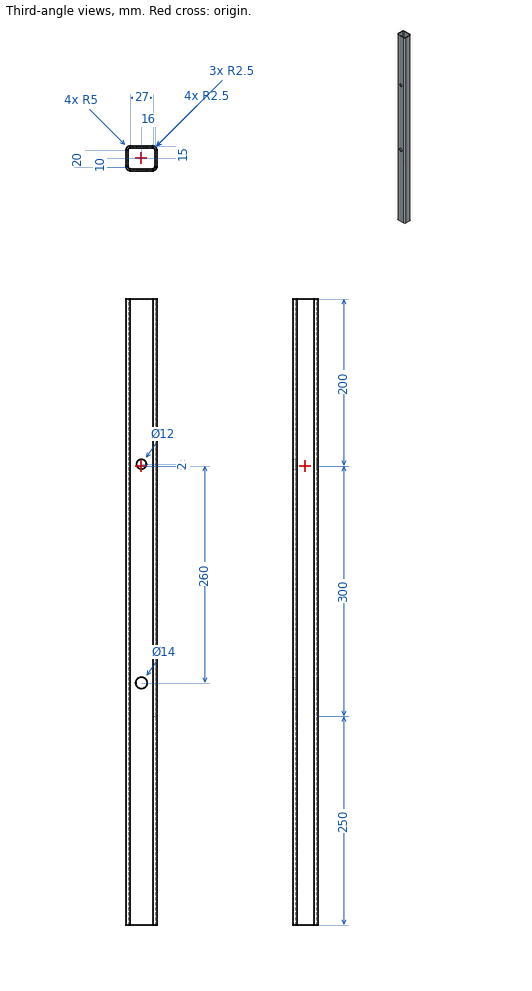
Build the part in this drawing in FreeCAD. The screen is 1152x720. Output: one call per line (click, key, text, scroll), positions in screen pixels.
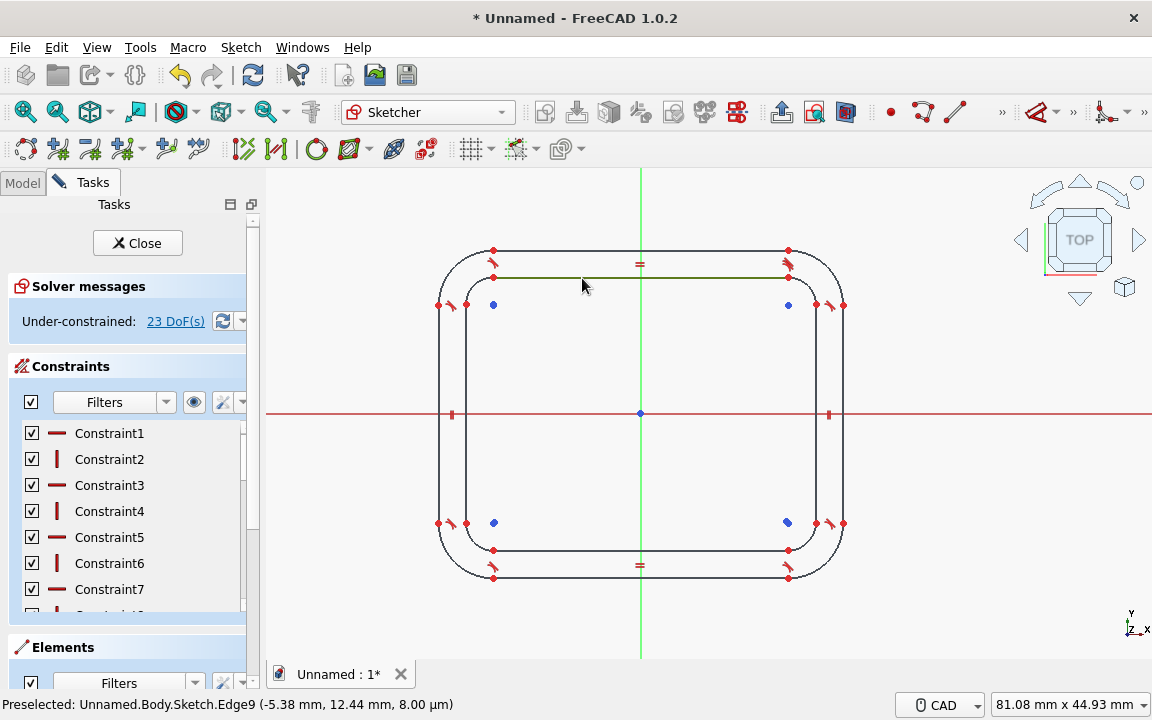
click(481, 281)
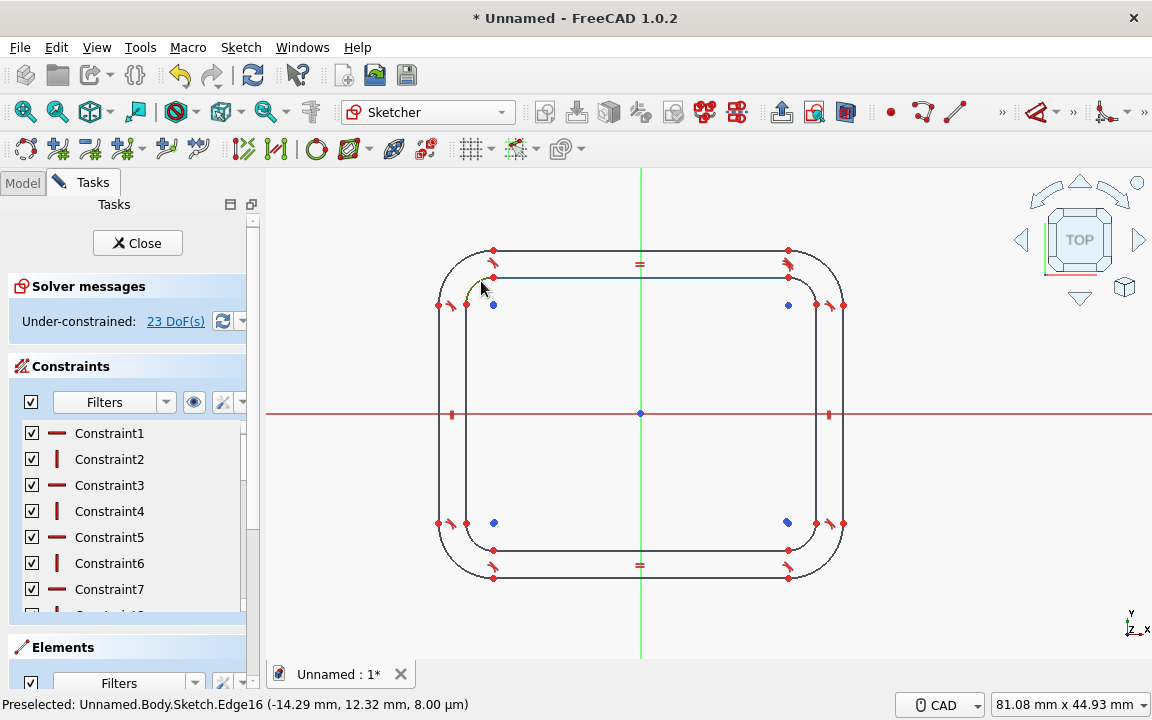
key(t)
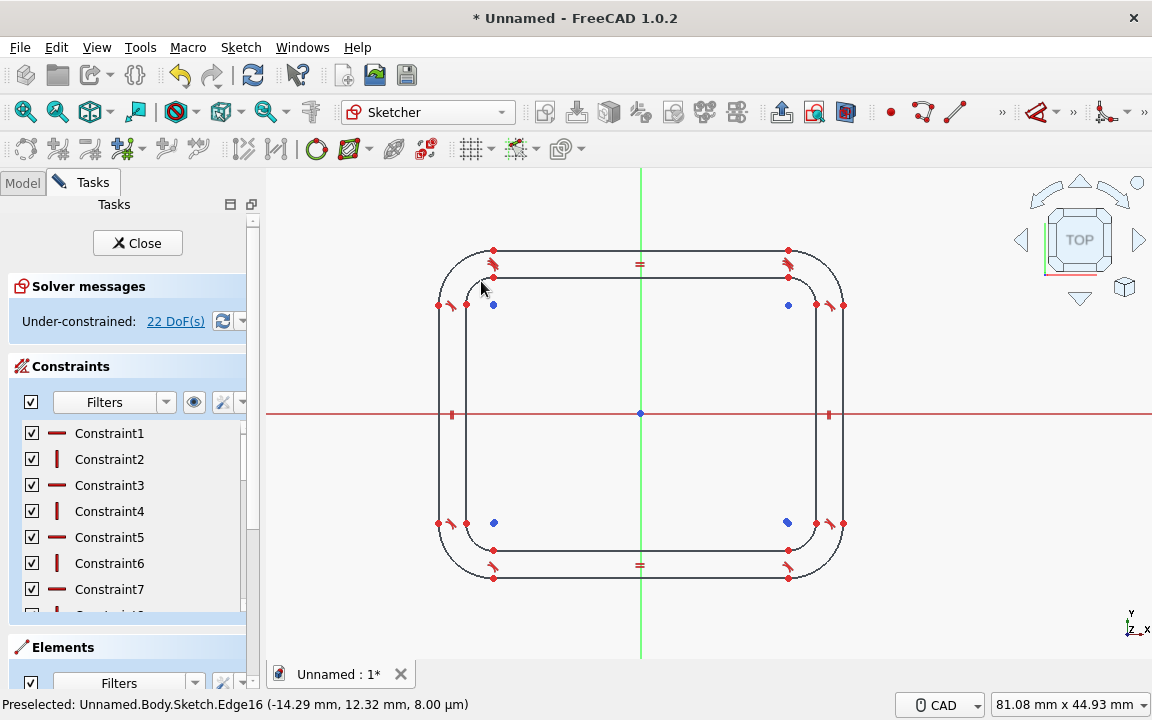
click(816, 371)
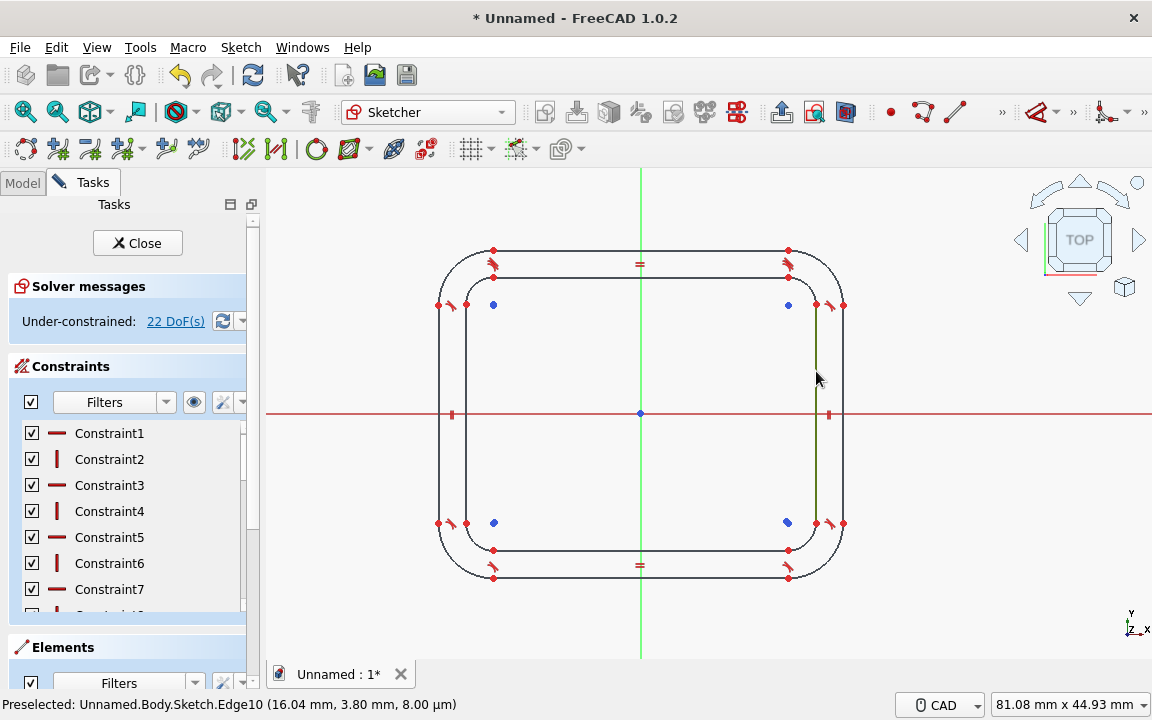
click(813, 292)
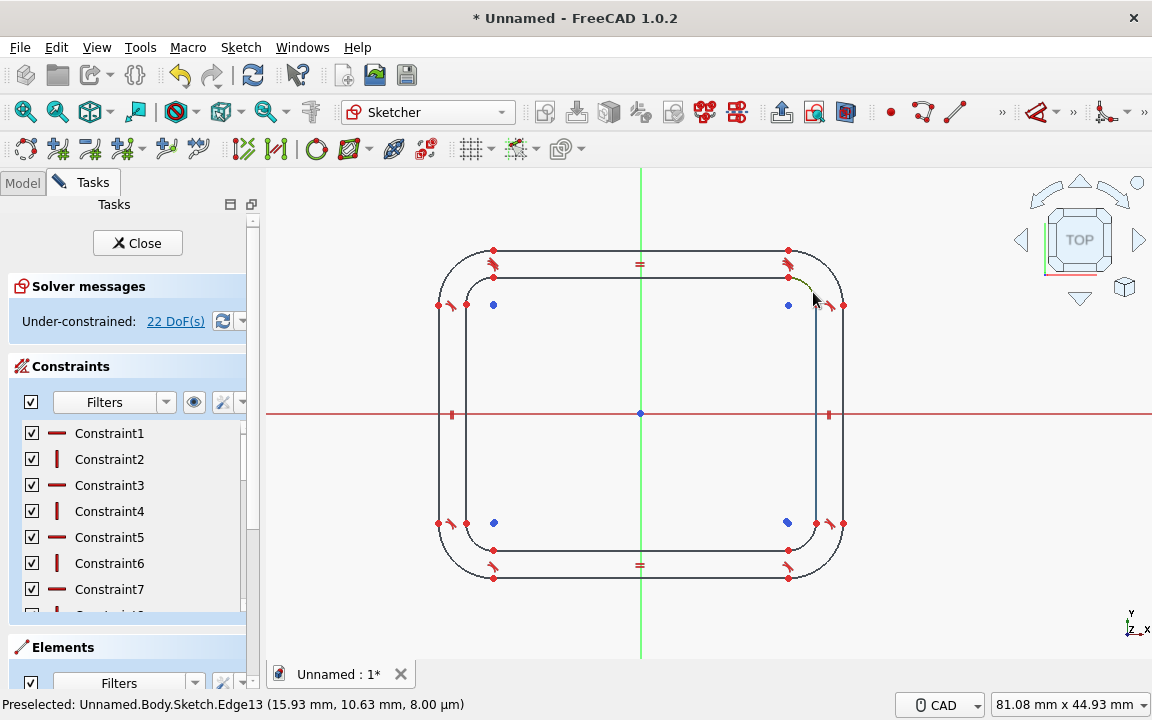
key(t)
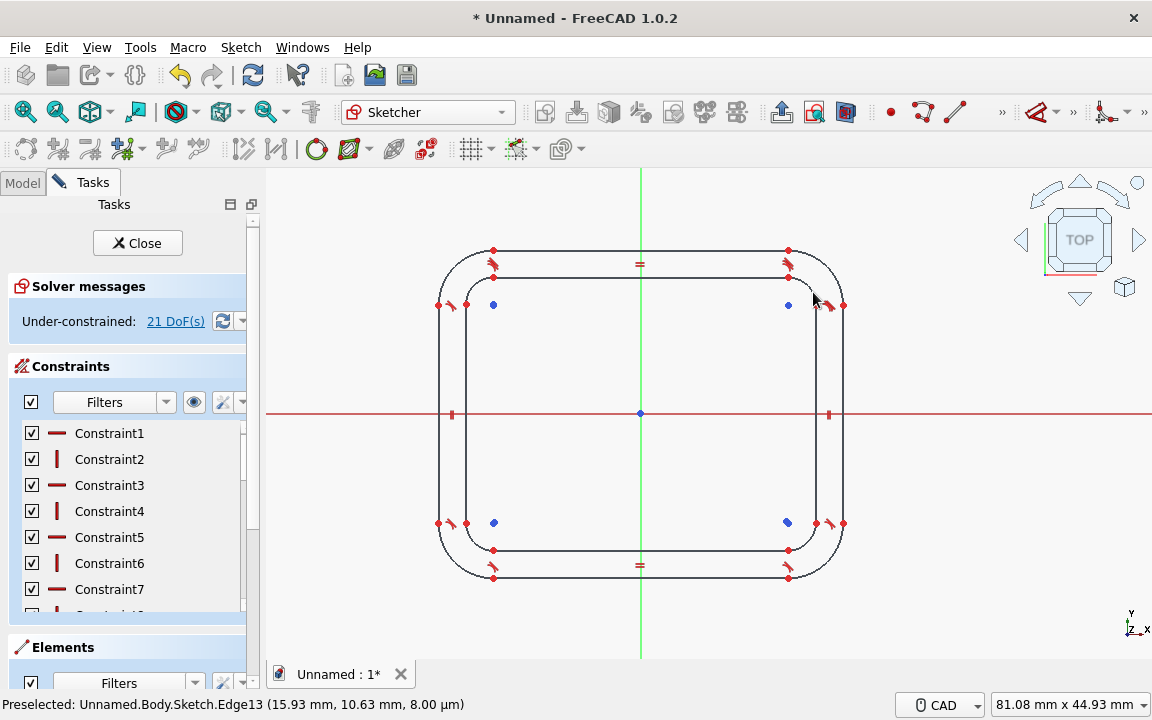
click(816, 371)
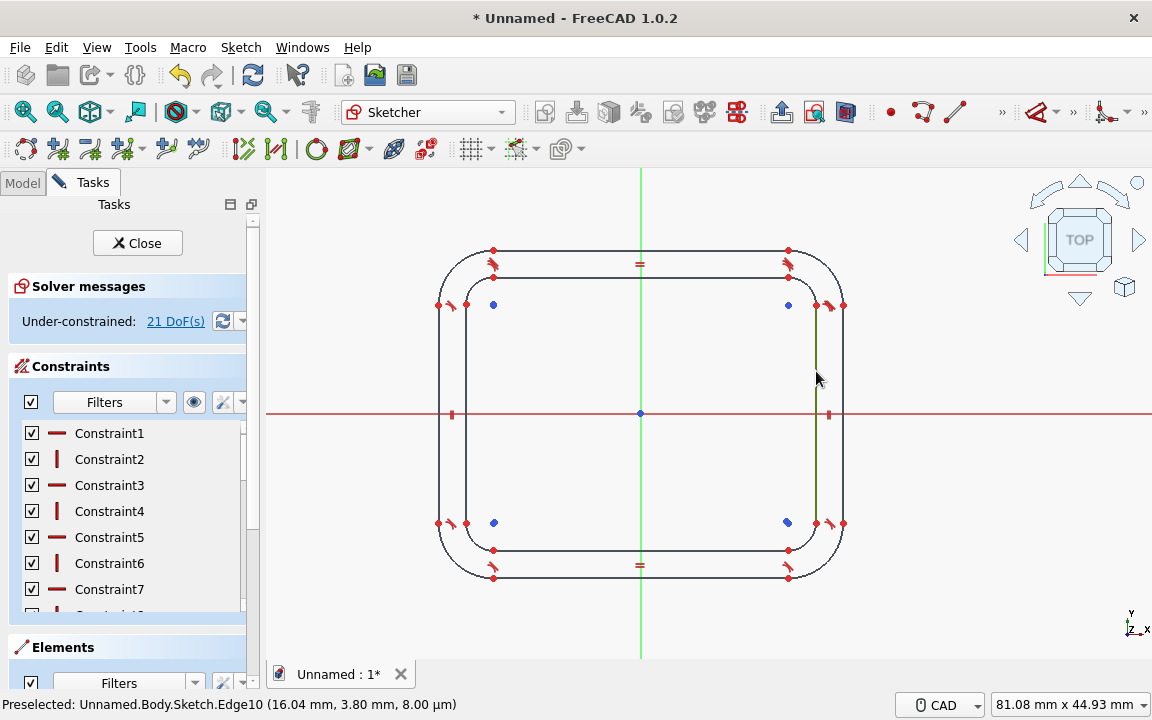
click(800, 548)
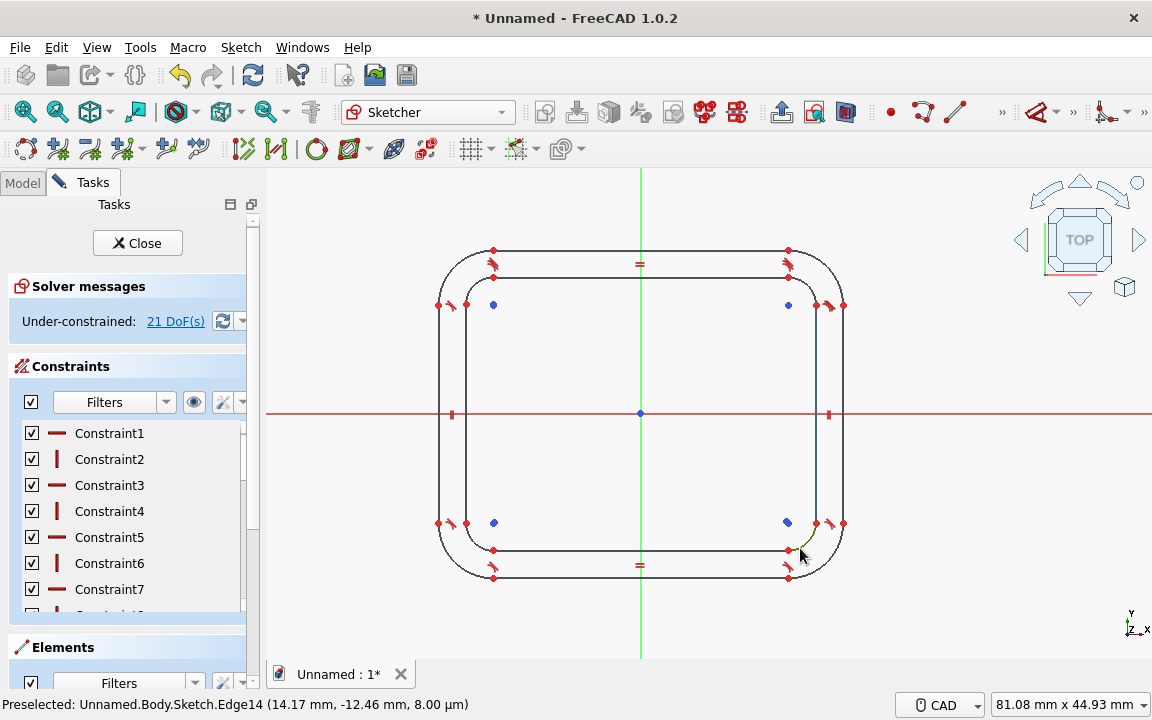
key(t)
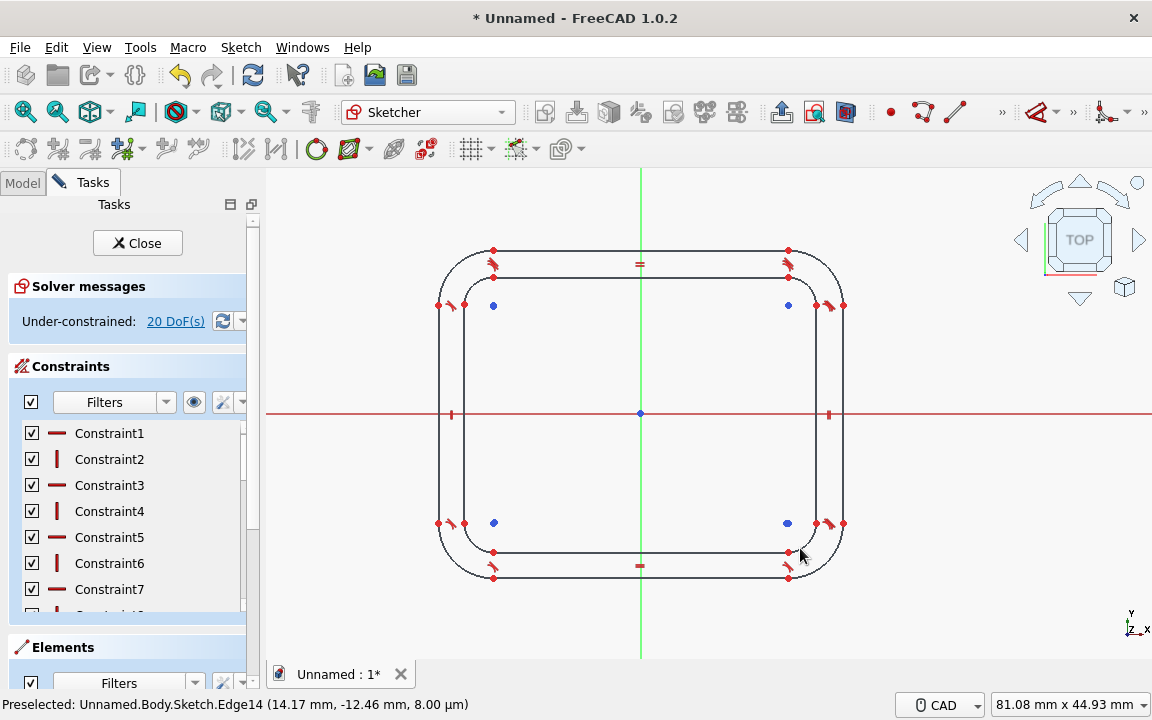
click(700, 553)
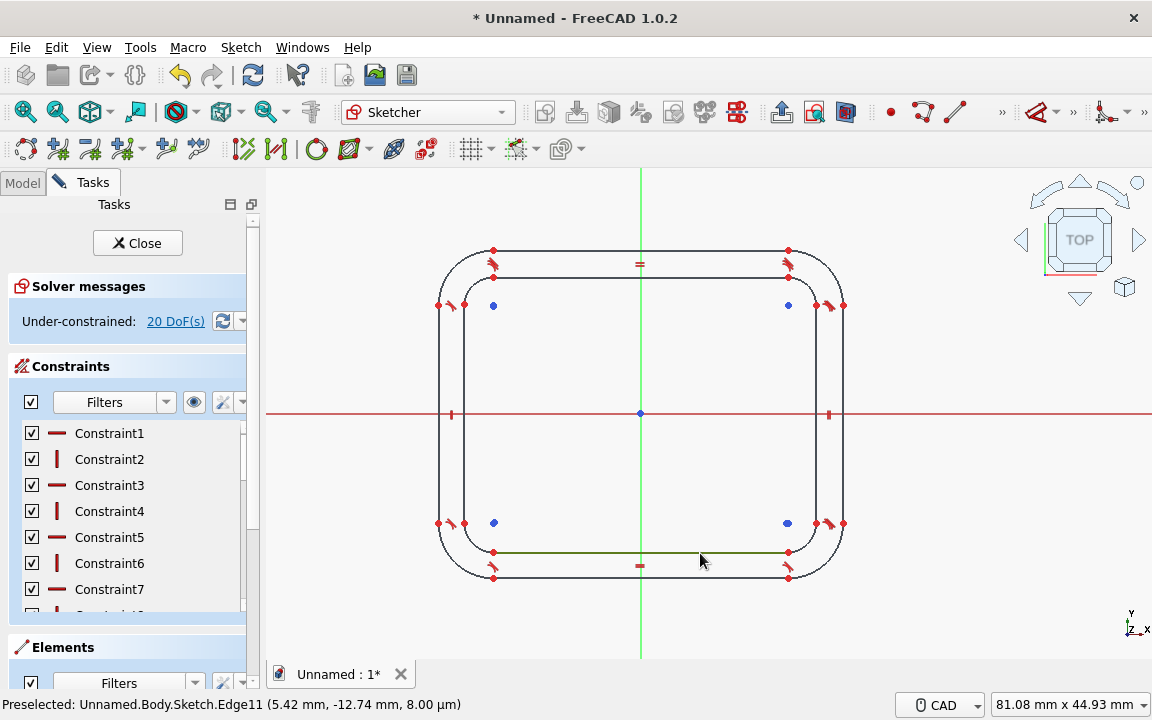
click(801, 549)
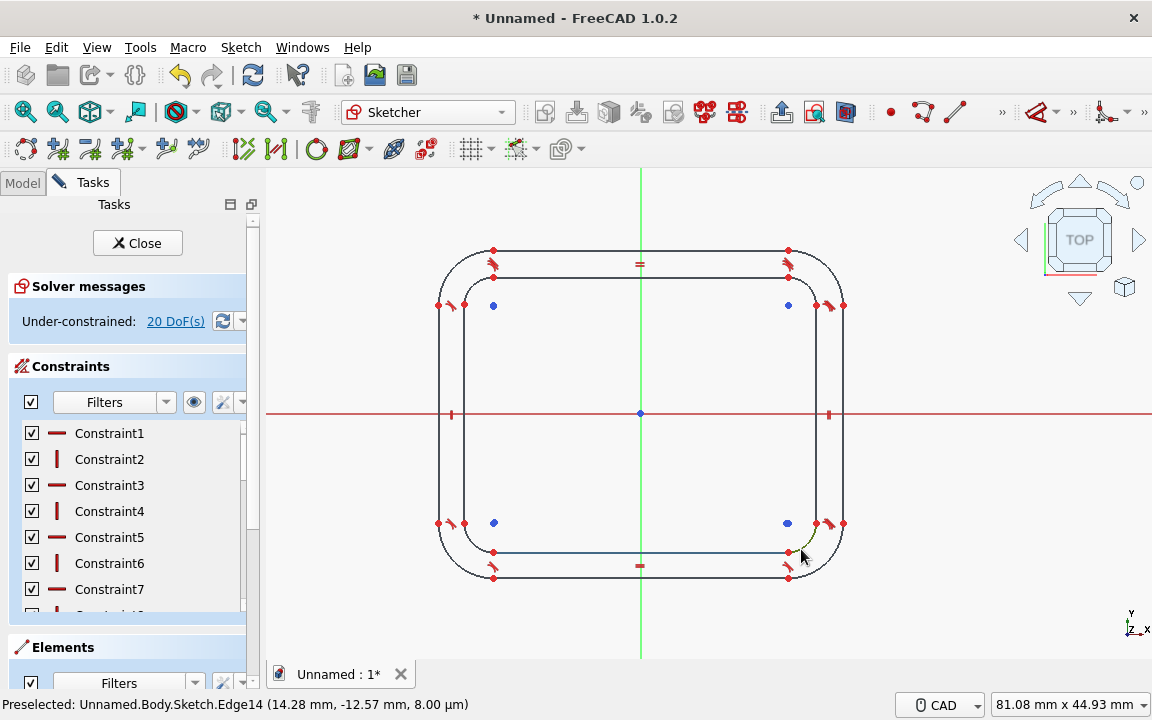
key(t)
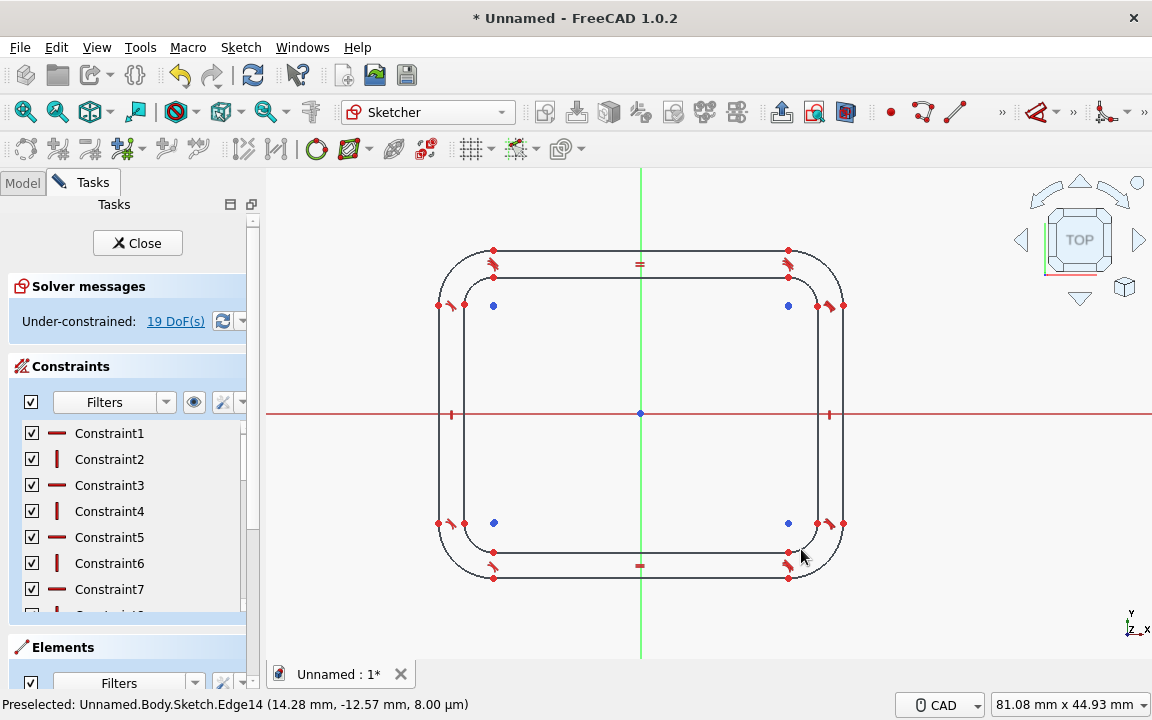
click(700, 553)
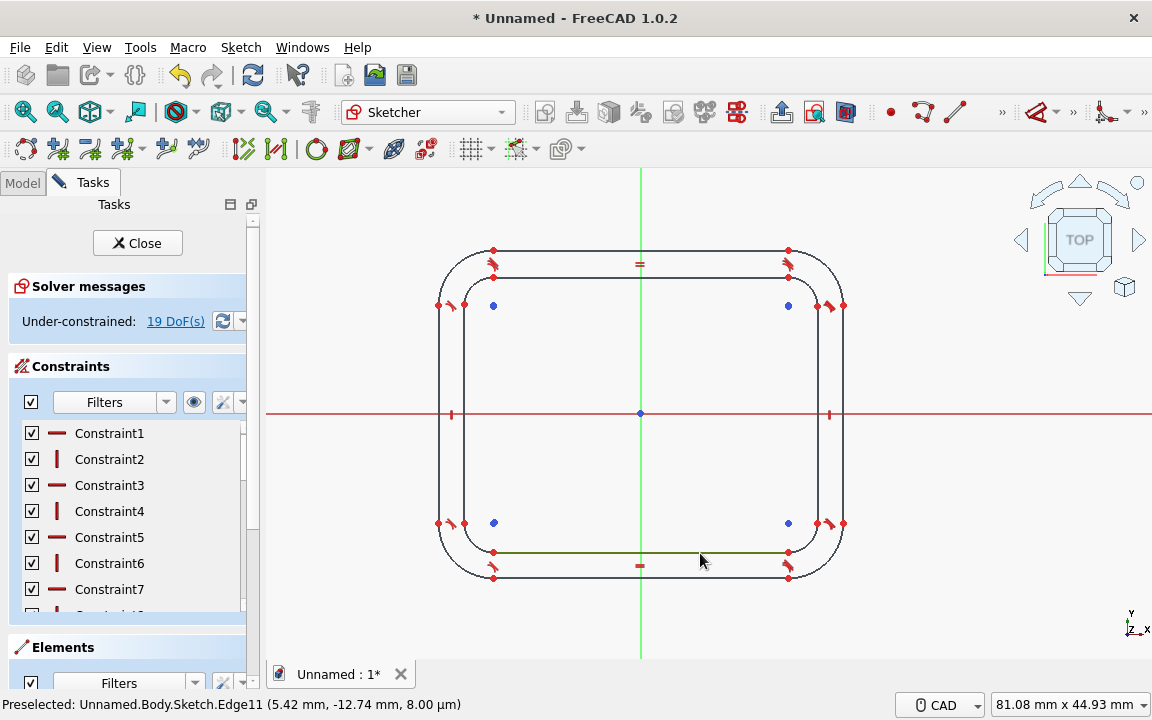
click(468, 537)